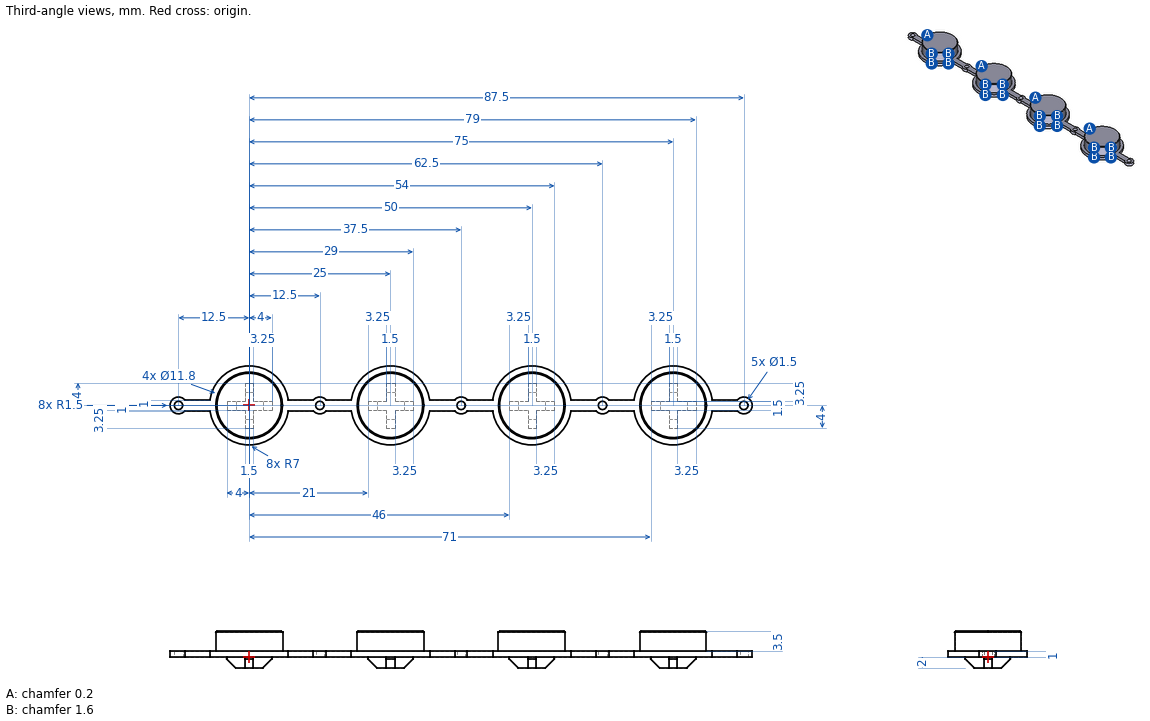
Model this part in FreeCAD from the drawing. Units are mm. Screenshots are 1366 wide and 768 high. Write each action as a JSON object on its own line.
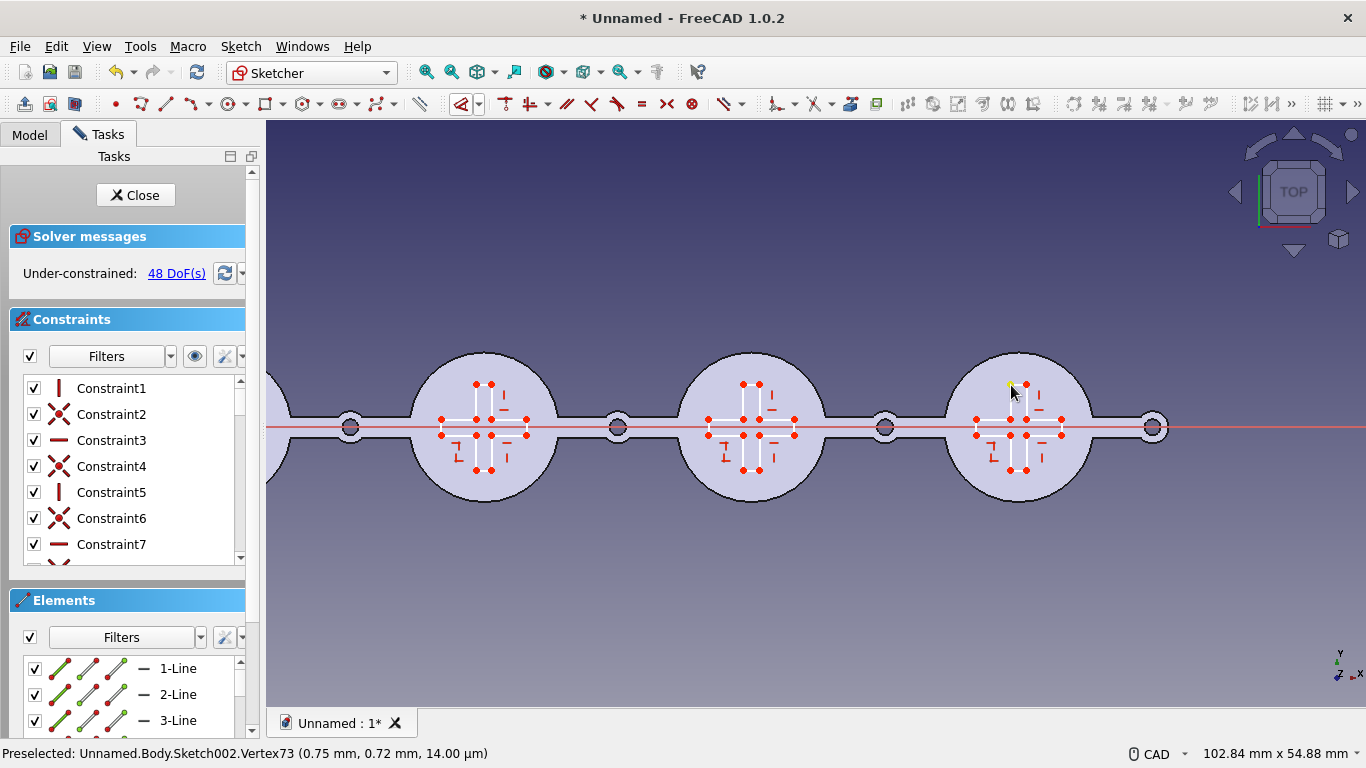
{"action": "left_click", "coordinate": [1011, 385]}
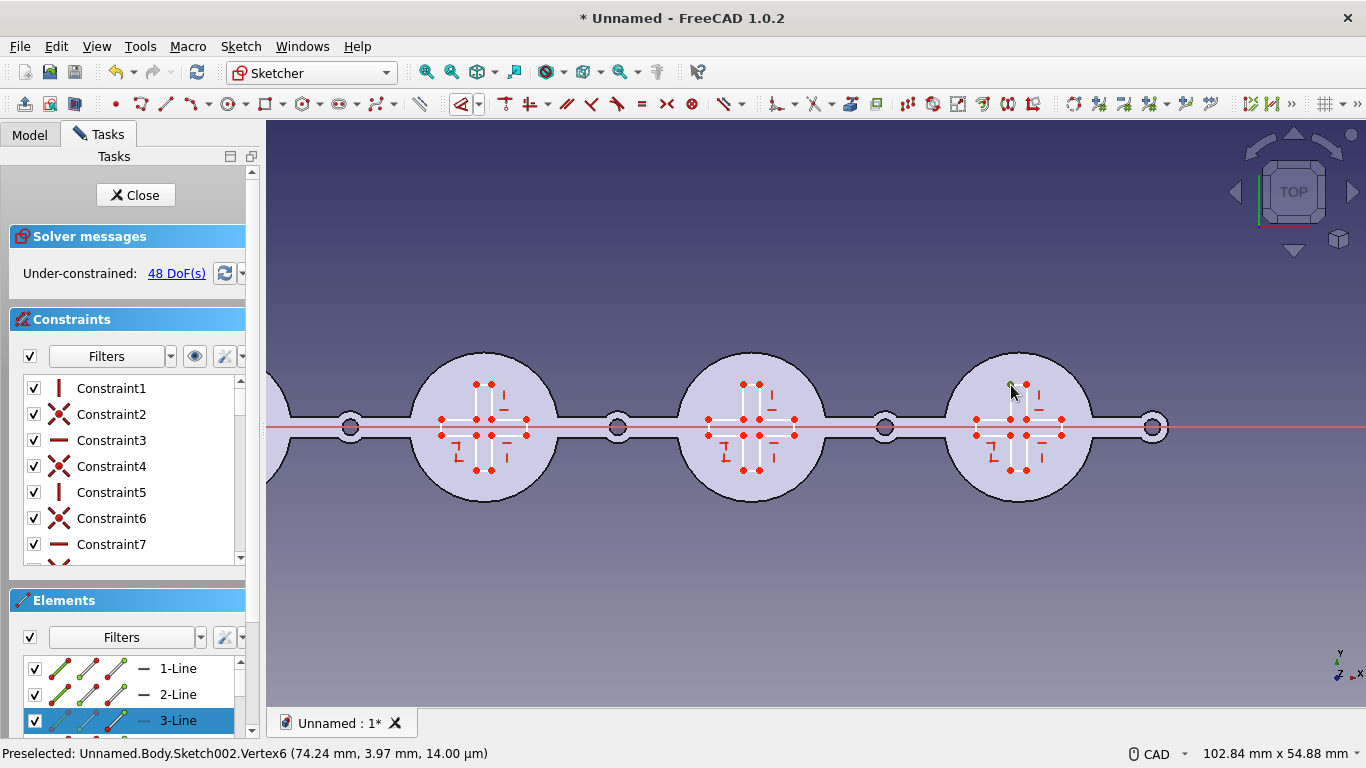
{"action": "left_click", "coordinate": [478, 104]}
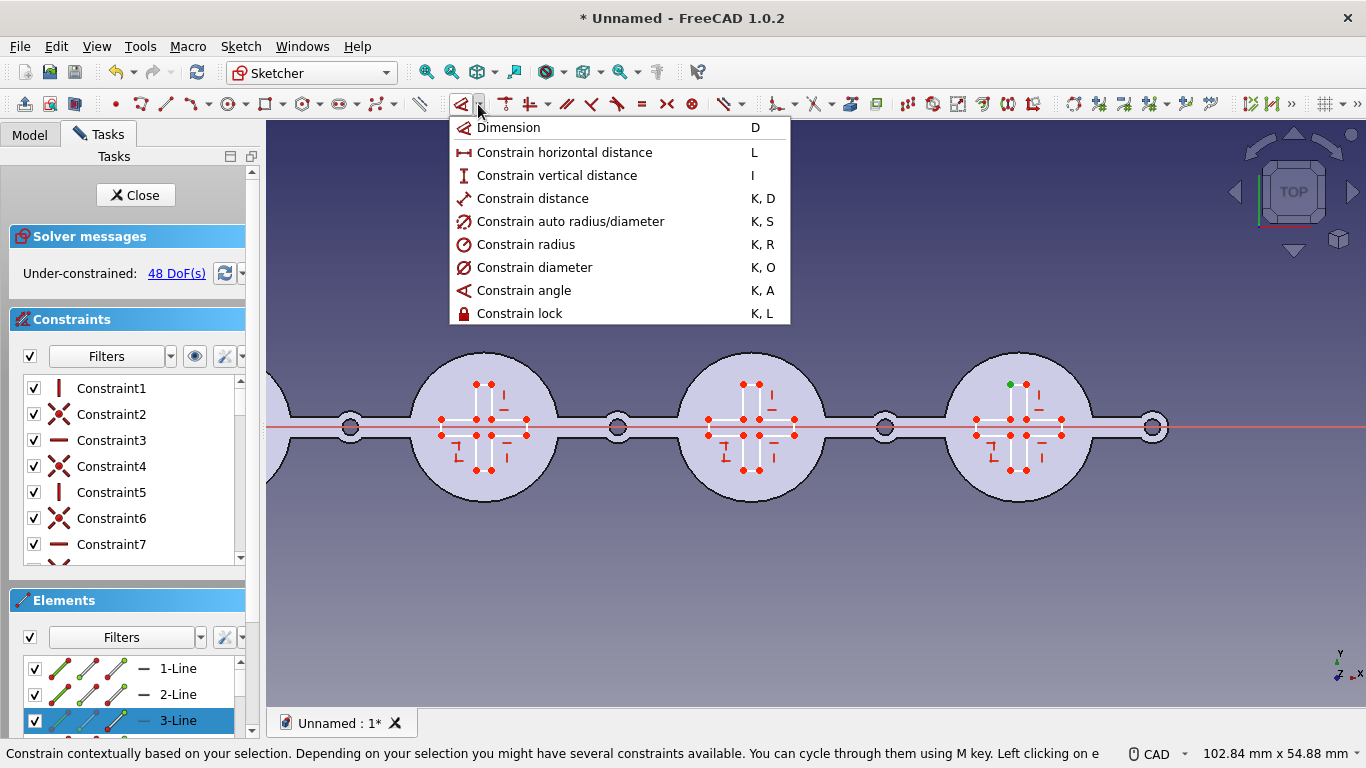
{"action": "left_click", "coordinate": [620, 176]}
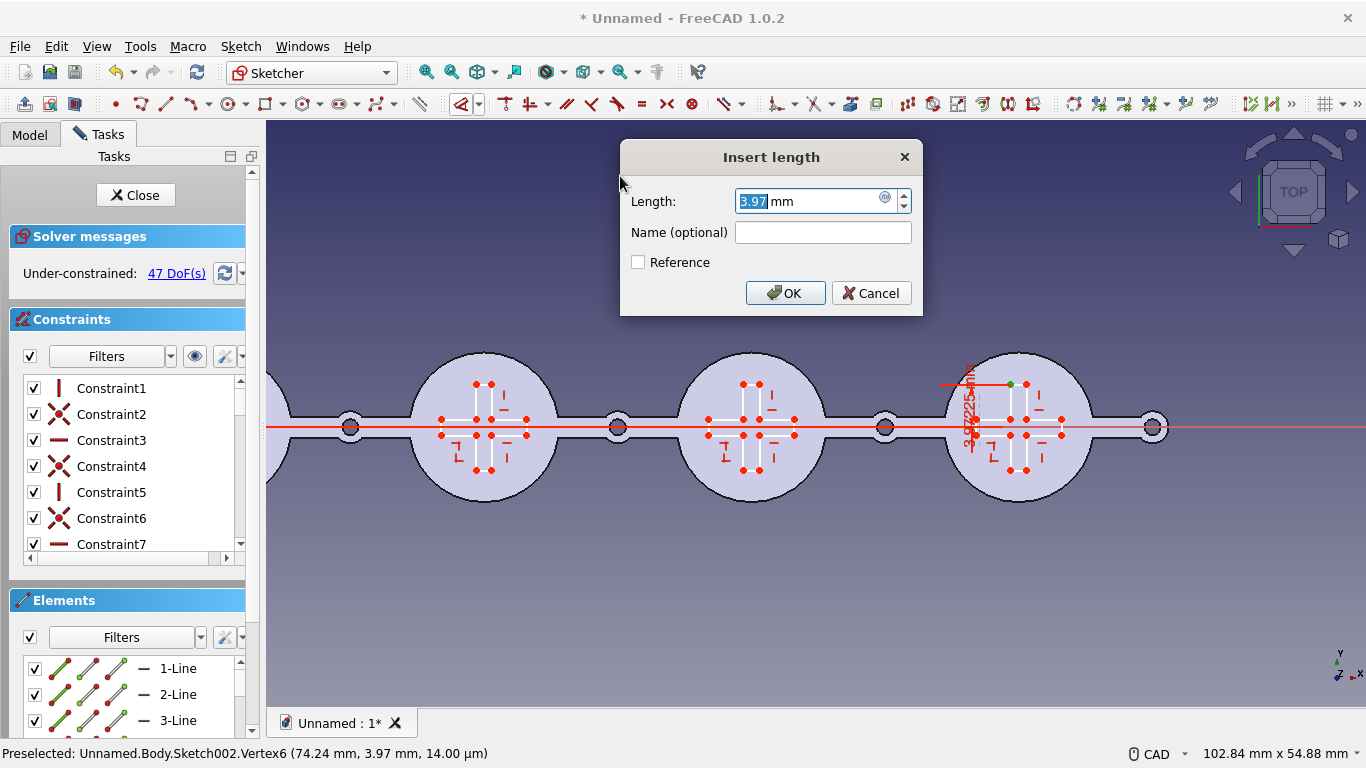
{"action": "type", "text": "4"}
{"action": "key", "text": "Return"}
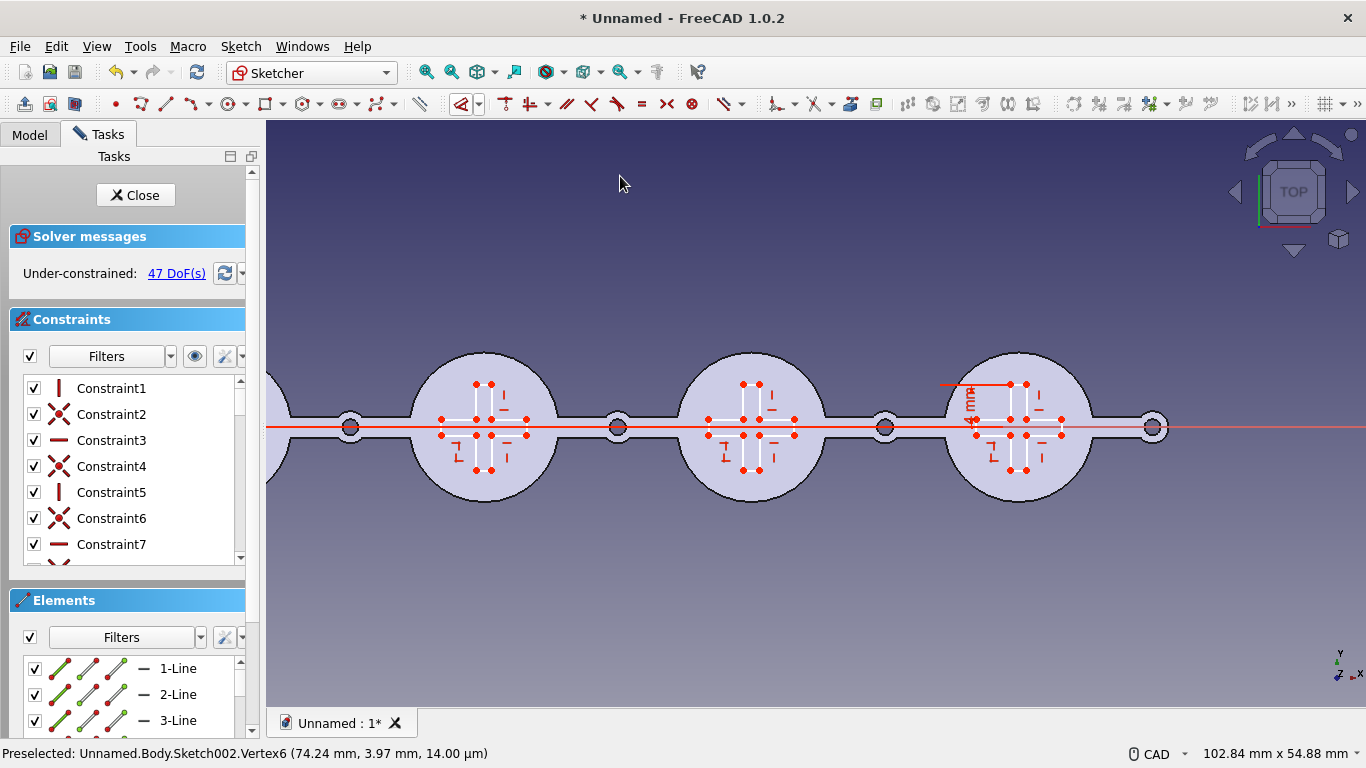
{"action": "left_click", "coordinate": [1027, 471]}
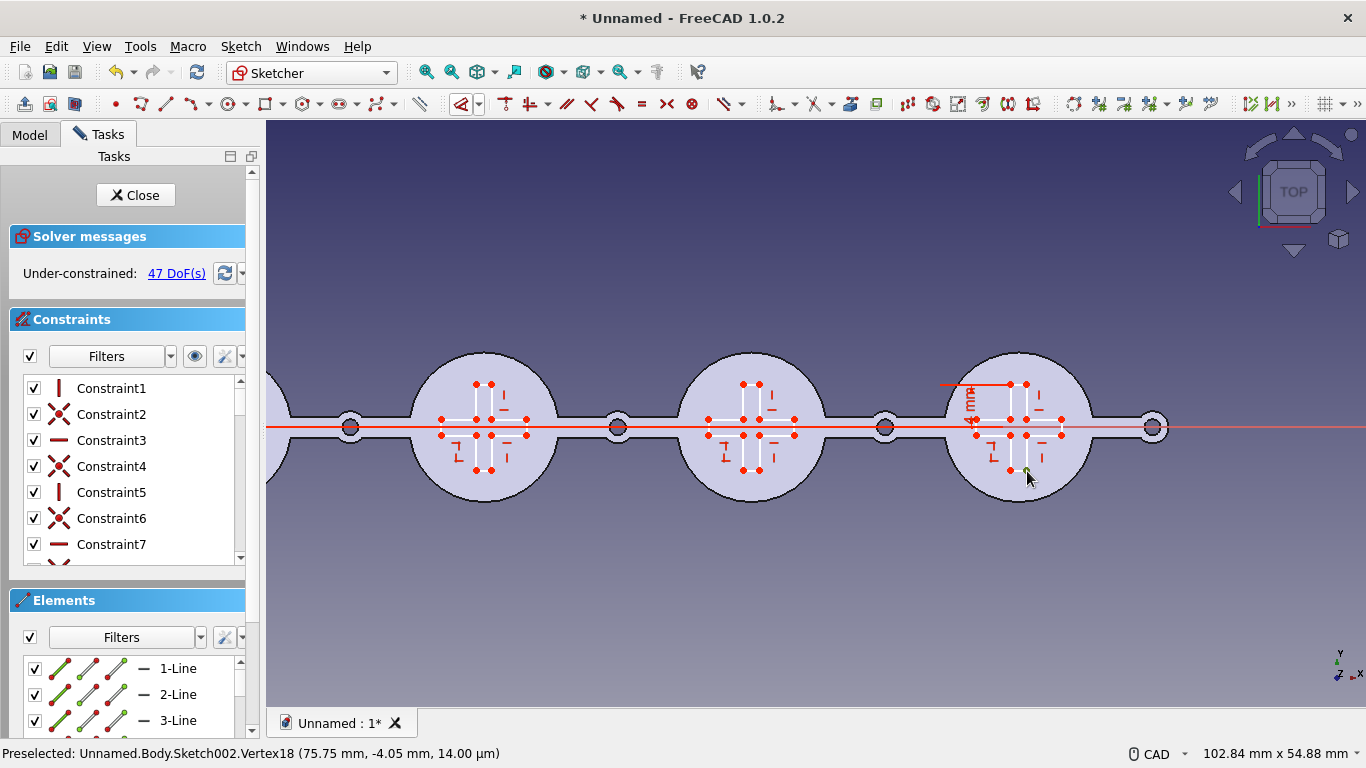
{"action": "key", "text": "i"}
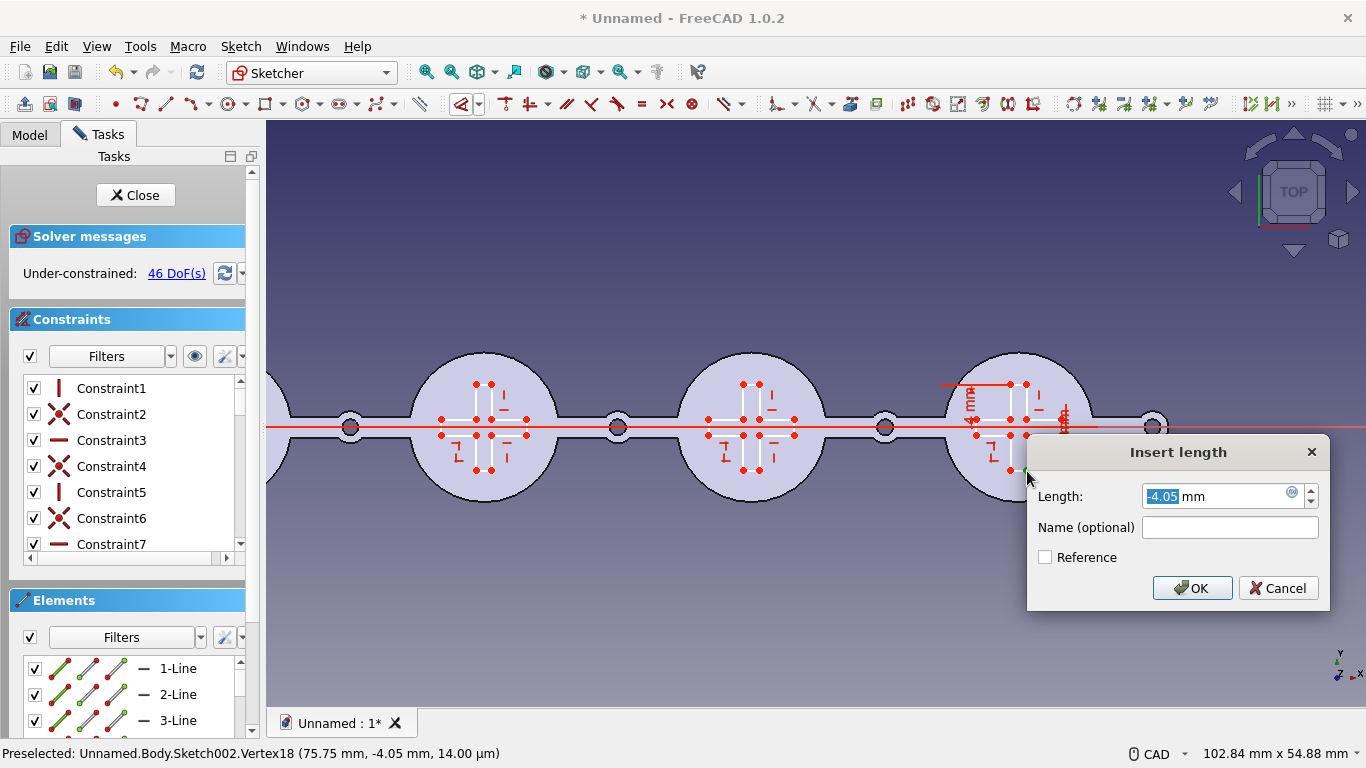
{"action": "type", "text": "-4"}
{"action": "key", "text": "Return"}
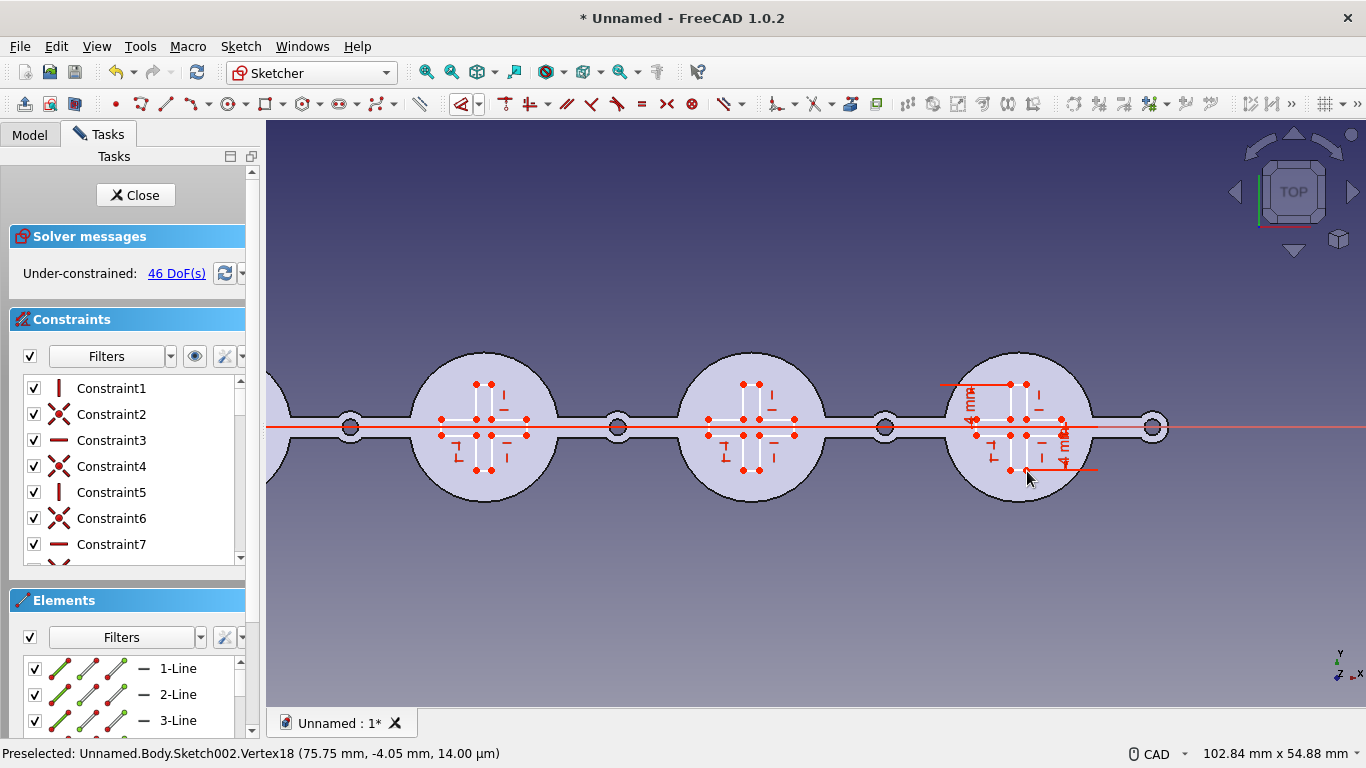
{"action": "left_click", "coordinate": [743, 385]}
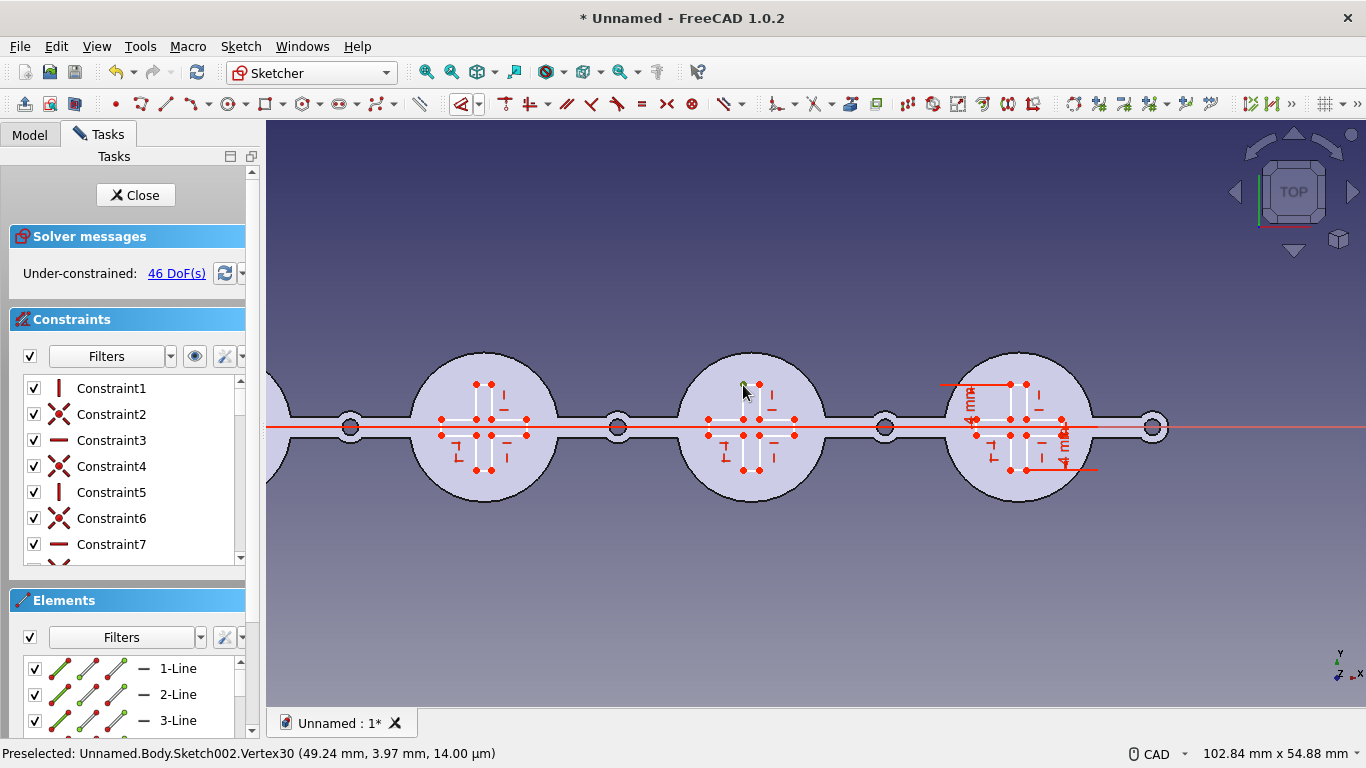
{"action": "key", "text": "i"}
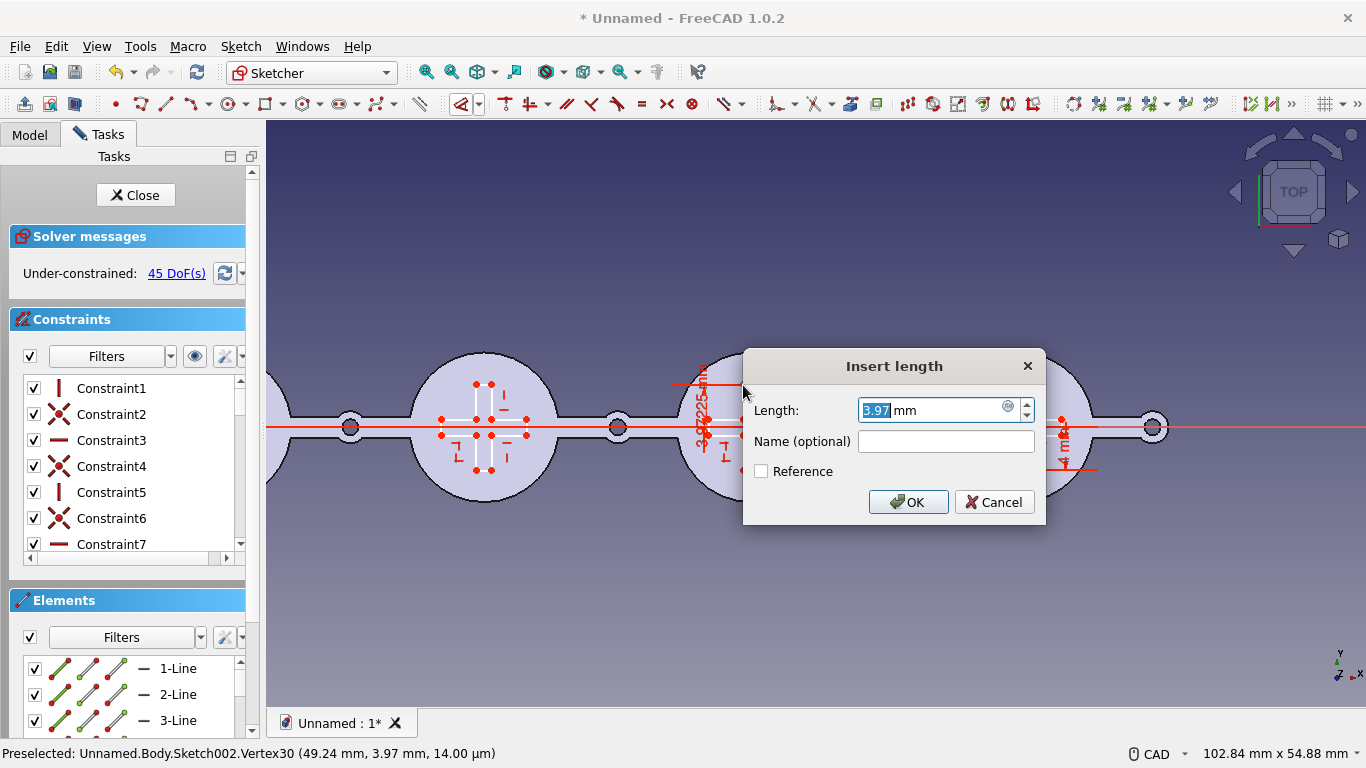
{"action": "type", "text": "4"}
{"action": "key", "text": "Return"}